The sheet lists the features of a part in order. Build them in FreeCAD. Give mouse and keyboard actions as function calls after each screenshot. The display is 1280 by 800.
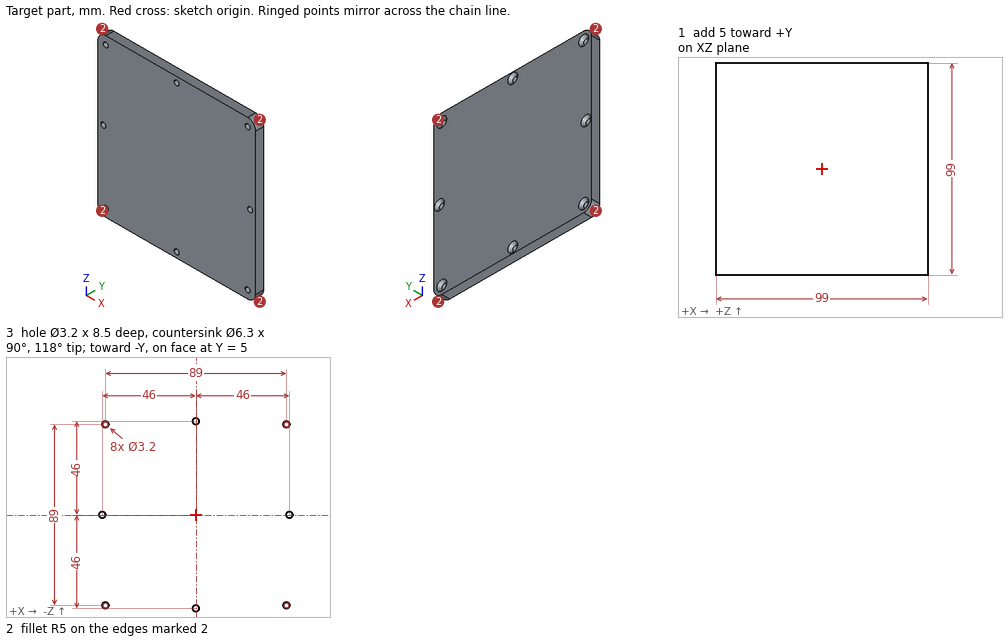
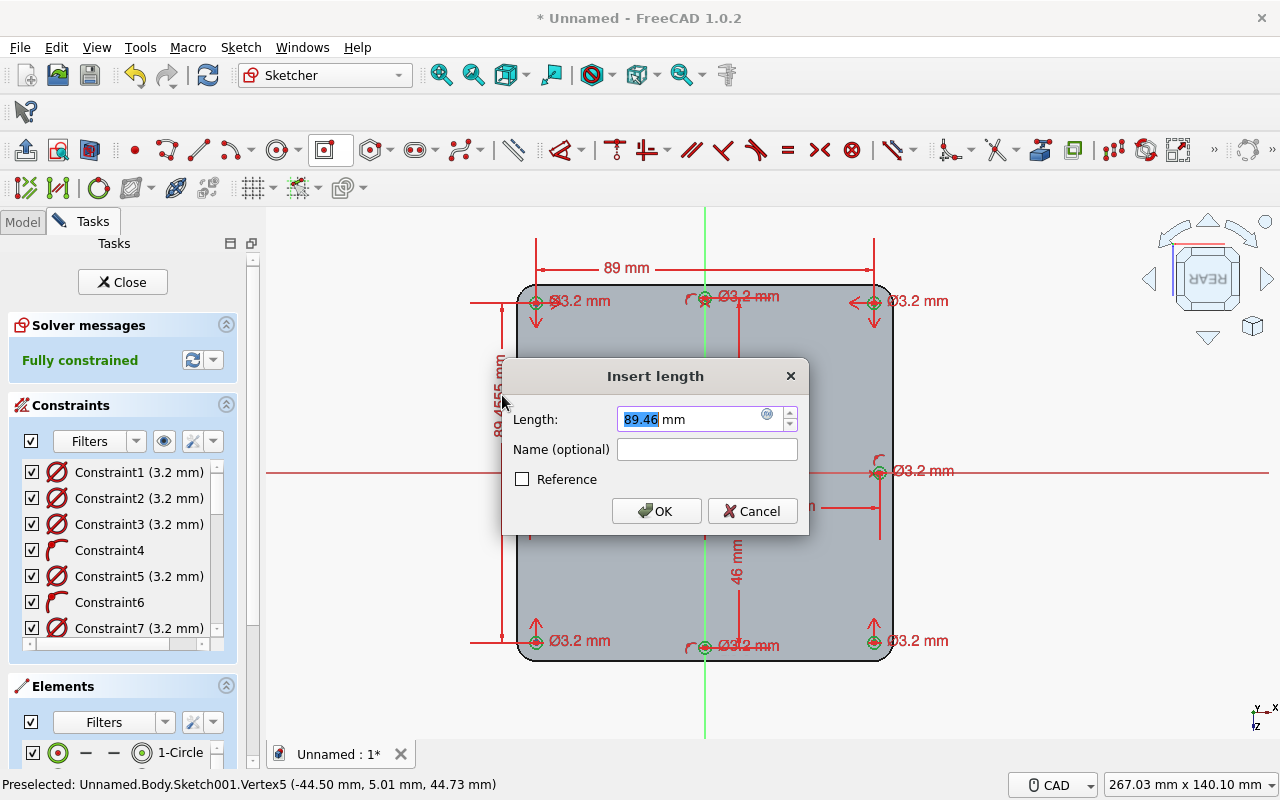
text(89)
key(Return)
key(Escape)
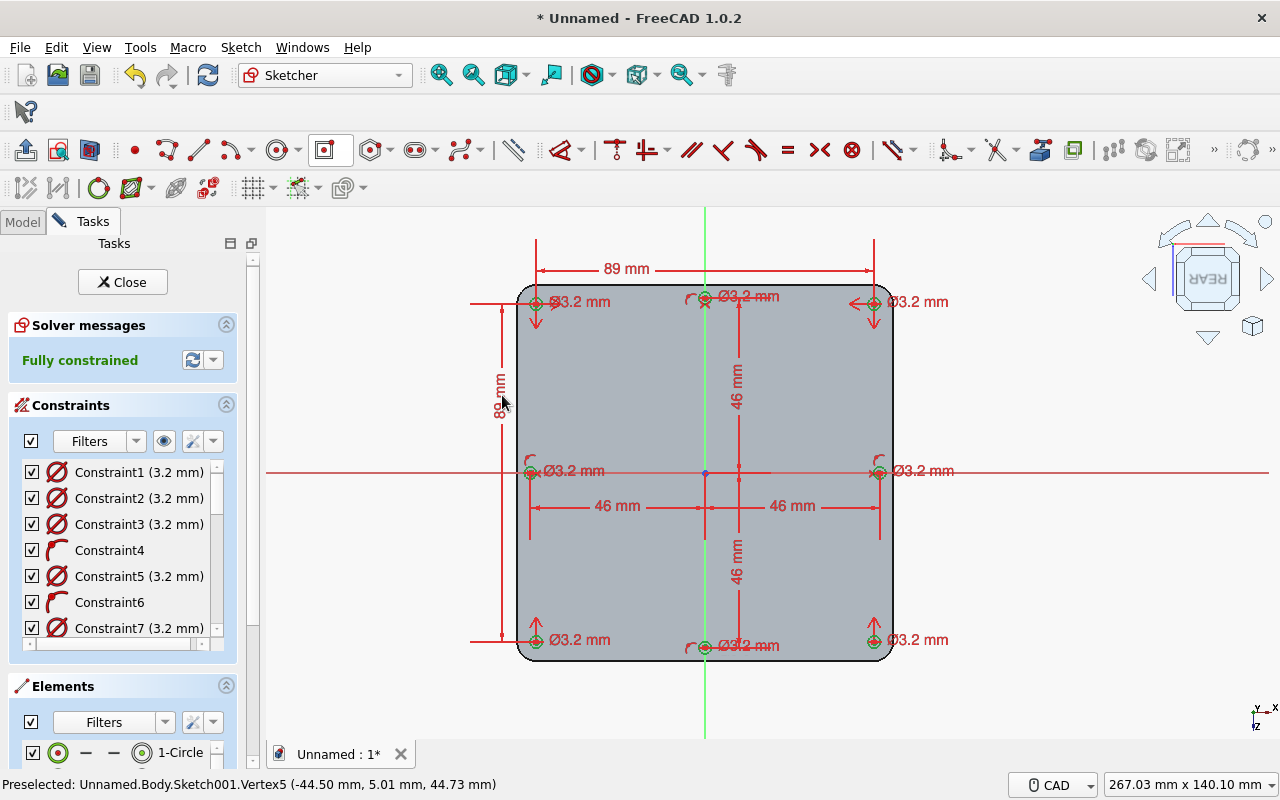
click(123, 282)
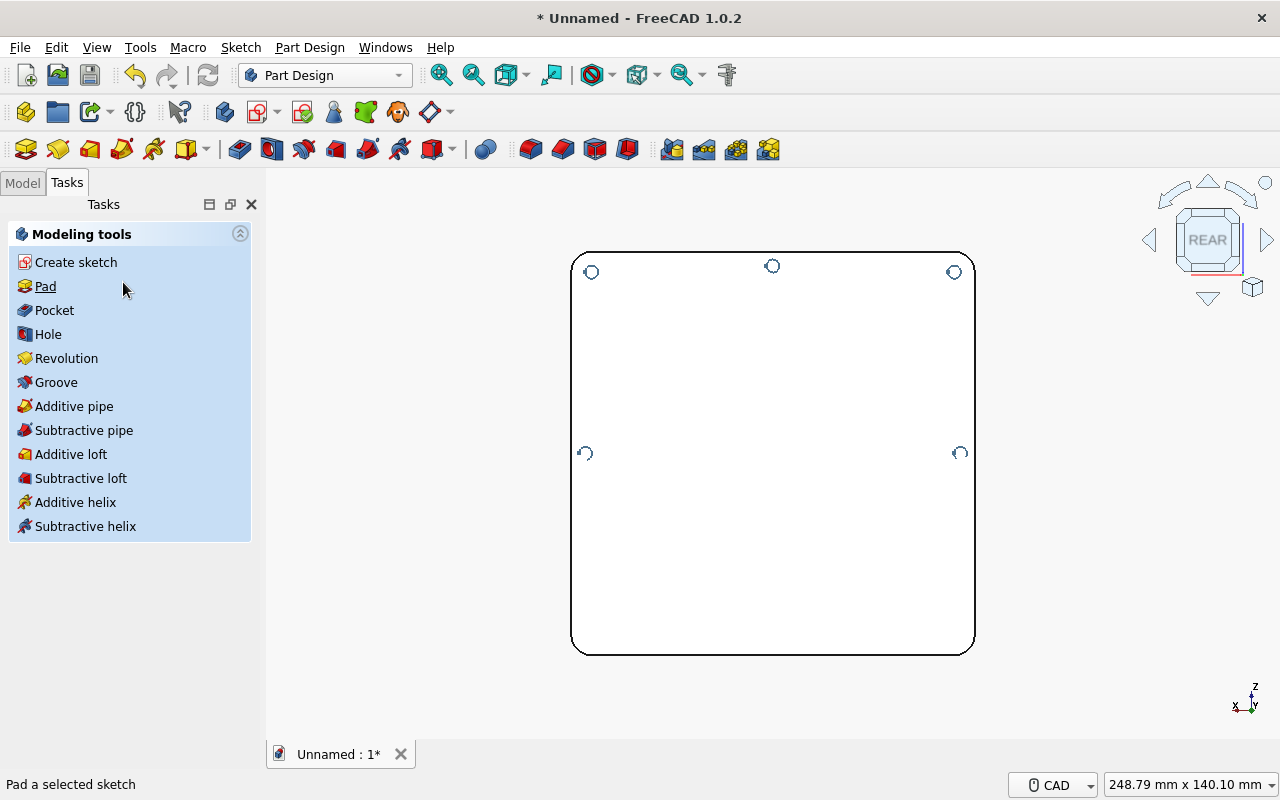
click(272, 150)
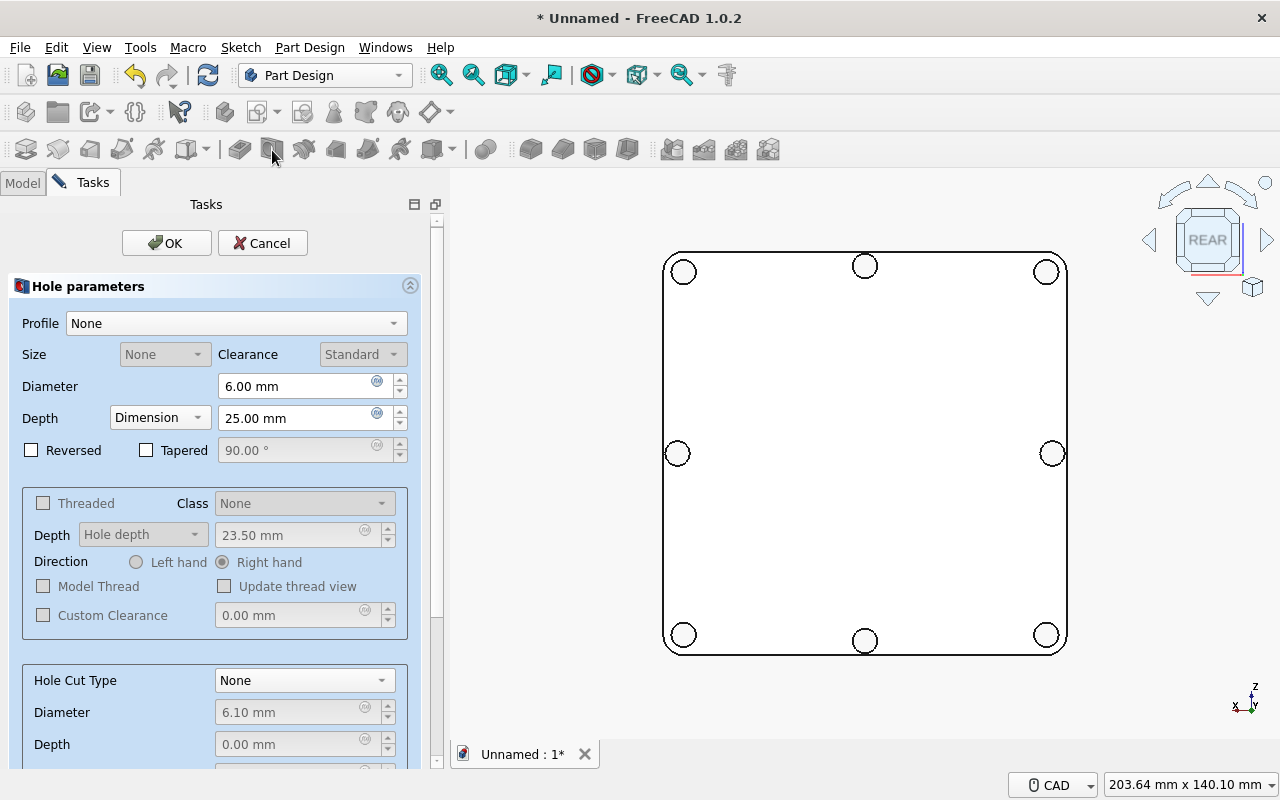
triple_click(305, 386)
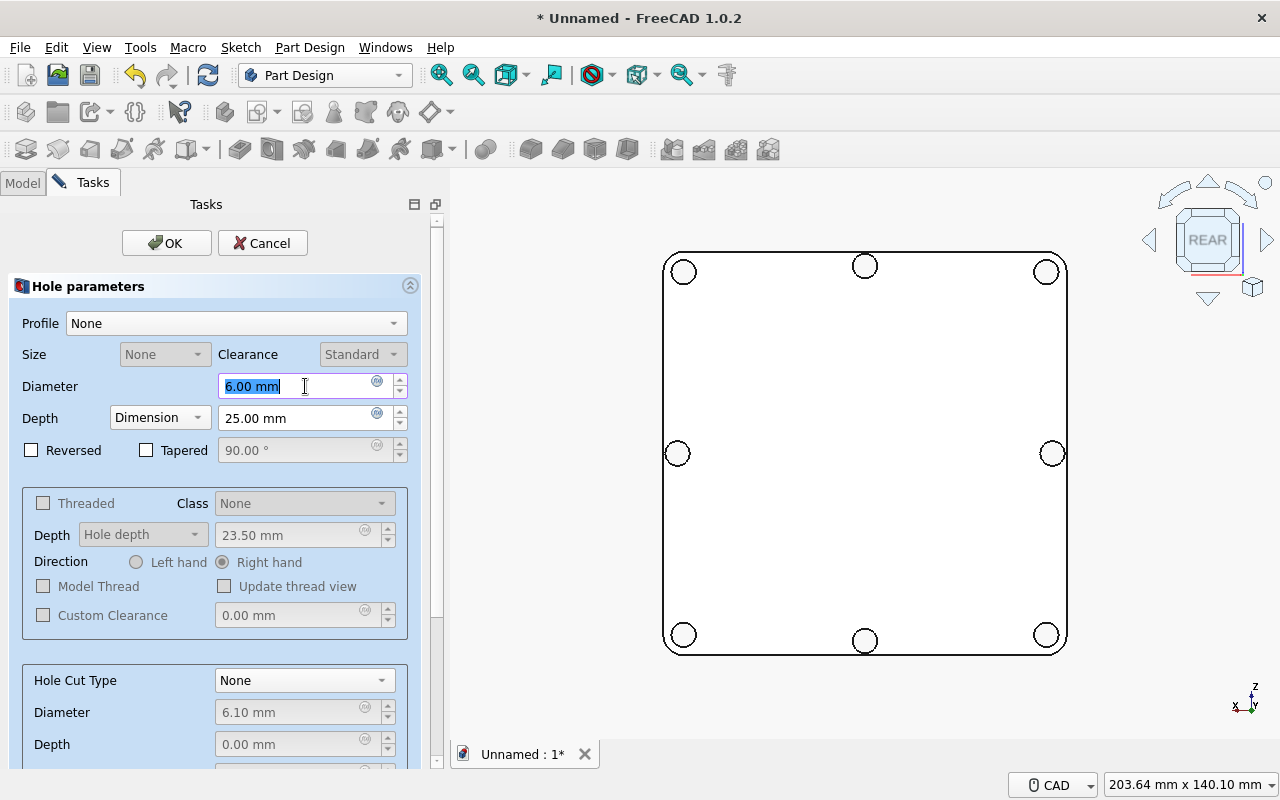
text(3.2)
key(Tab)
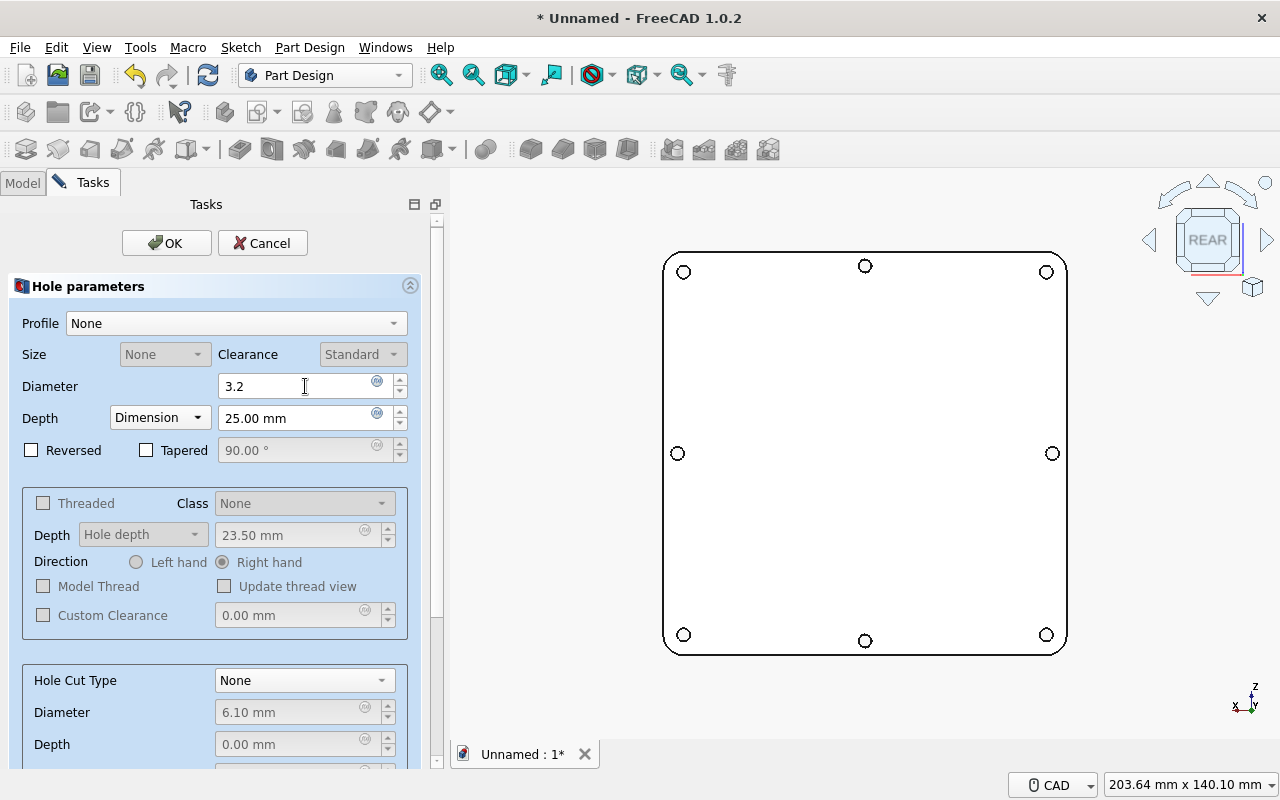
triple_click(305, 418)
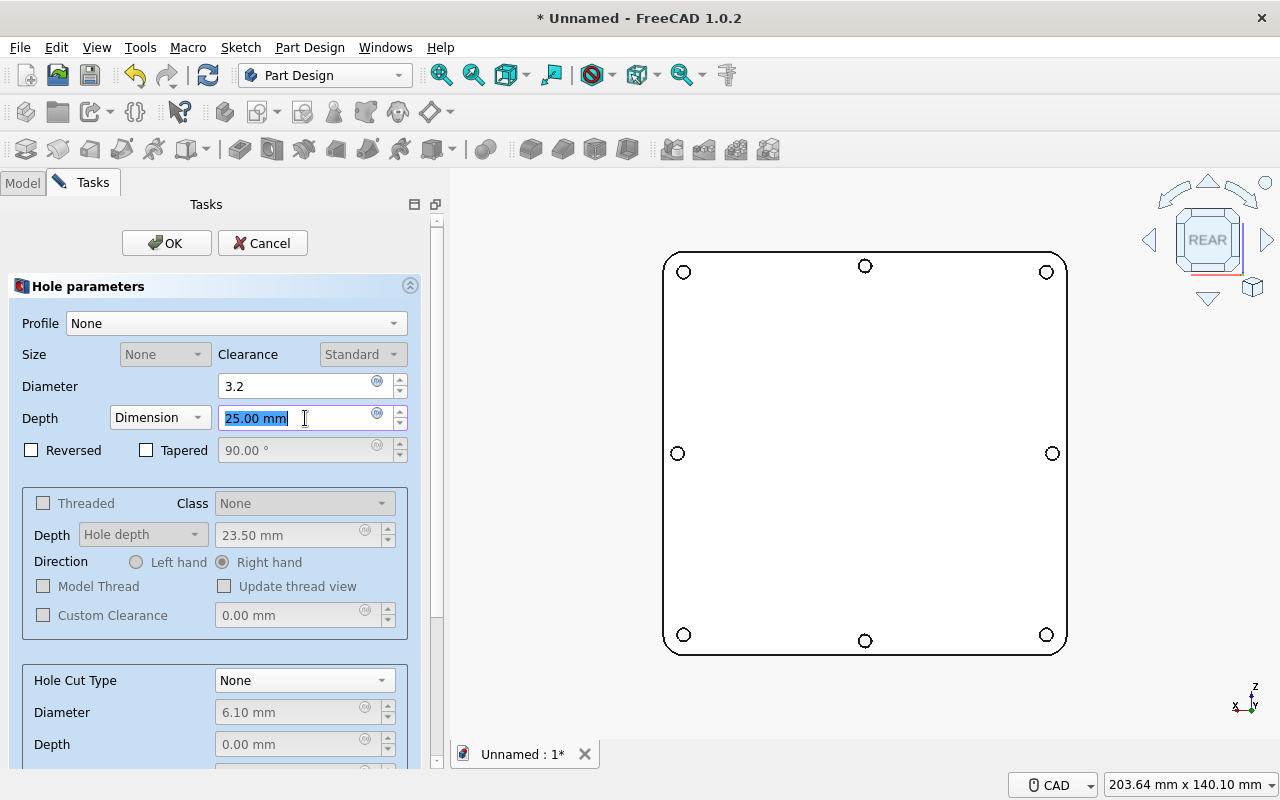
text(8.5)
key(Tab)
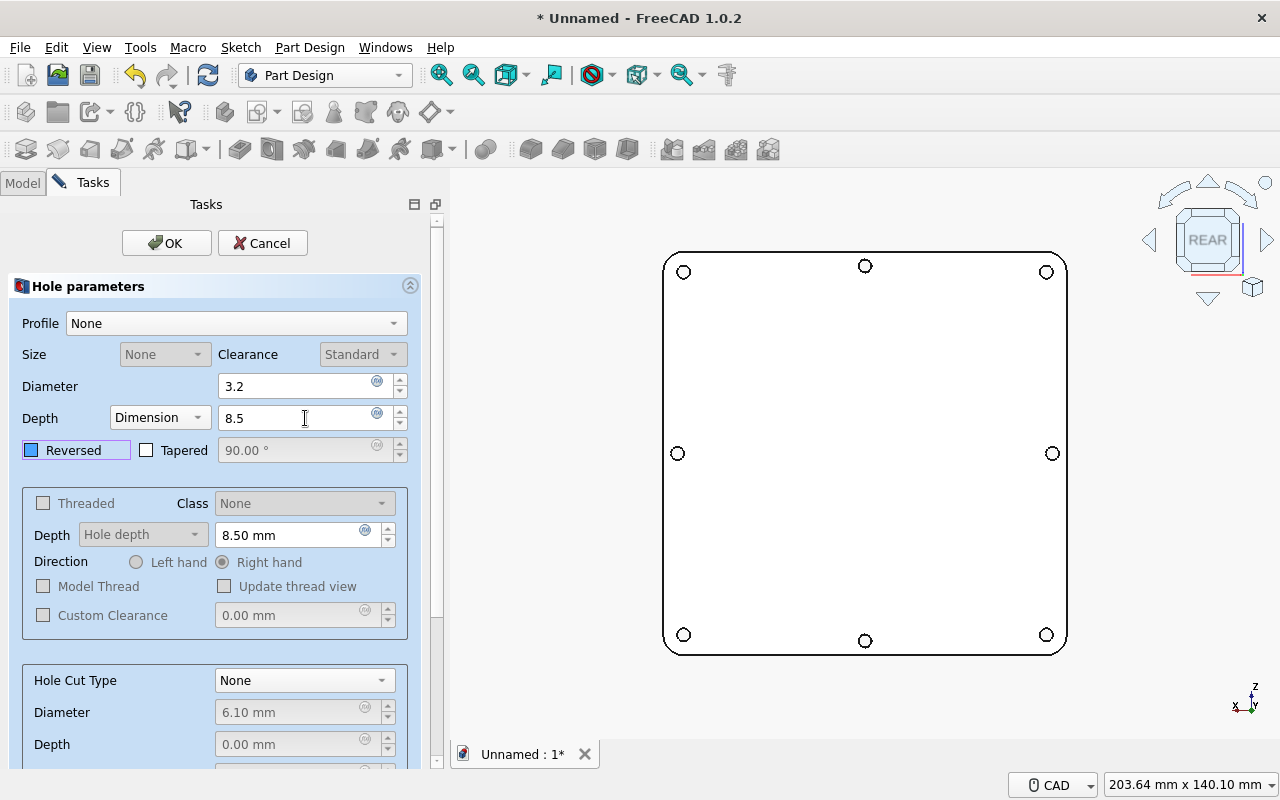
click(306, 680)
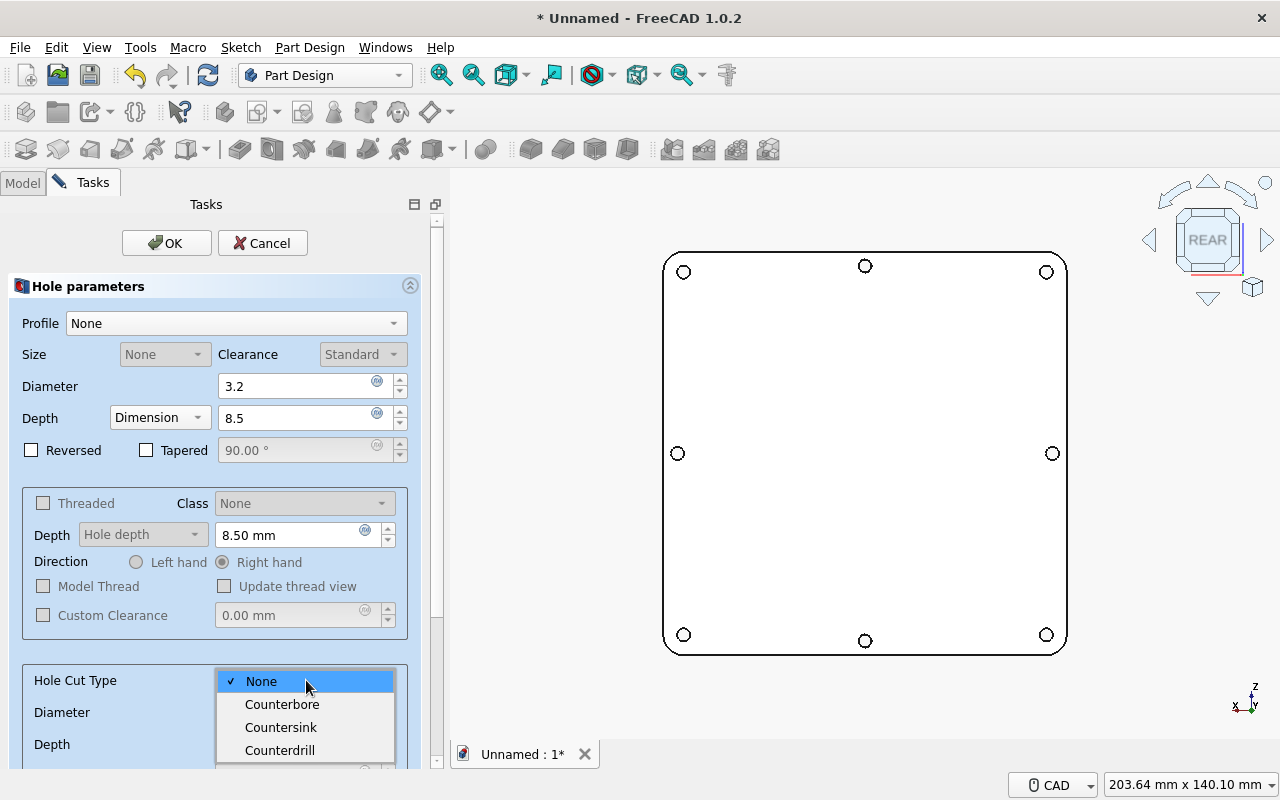
click(304, 728)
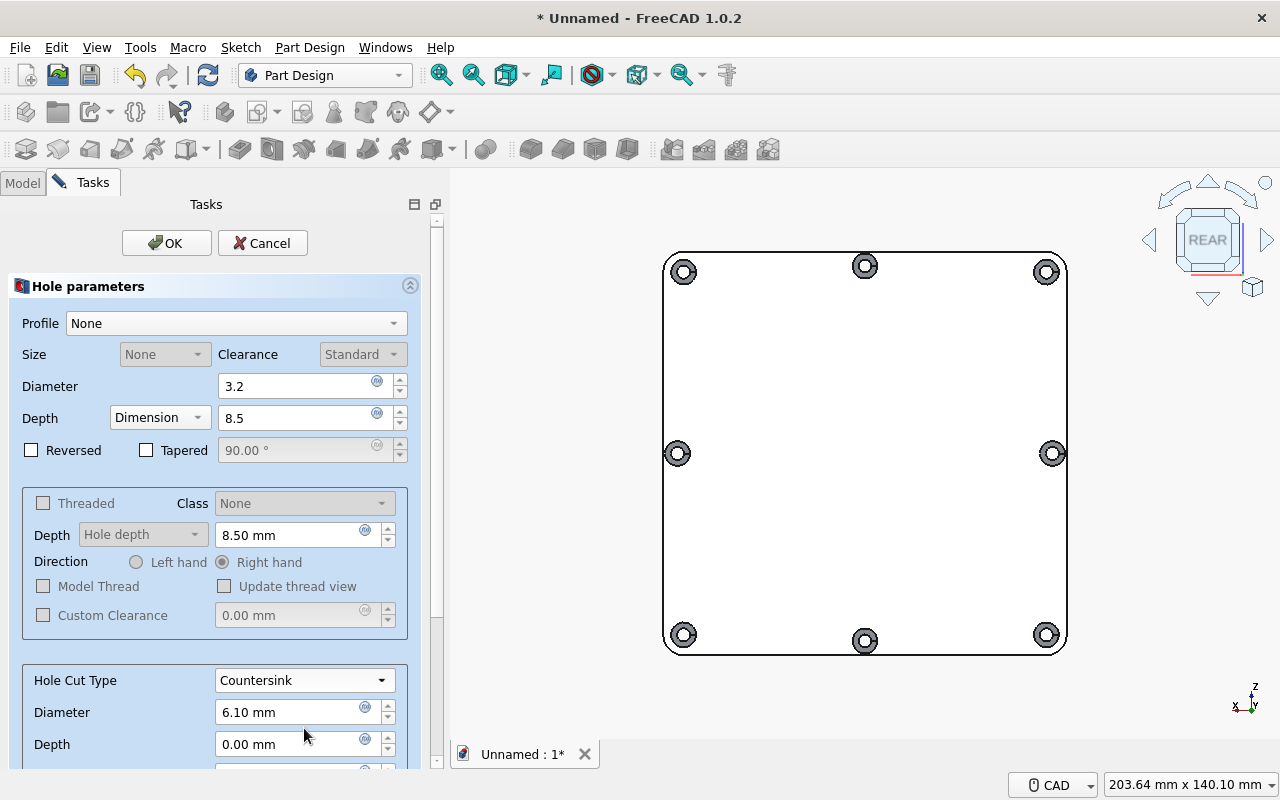
triple_click(298, 712)